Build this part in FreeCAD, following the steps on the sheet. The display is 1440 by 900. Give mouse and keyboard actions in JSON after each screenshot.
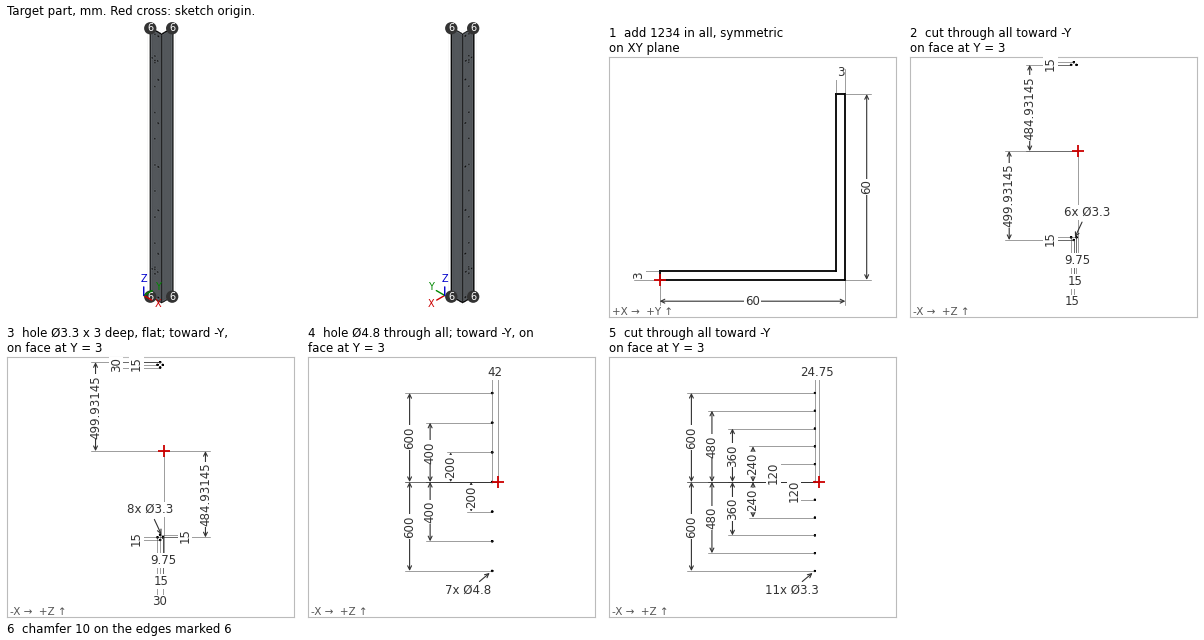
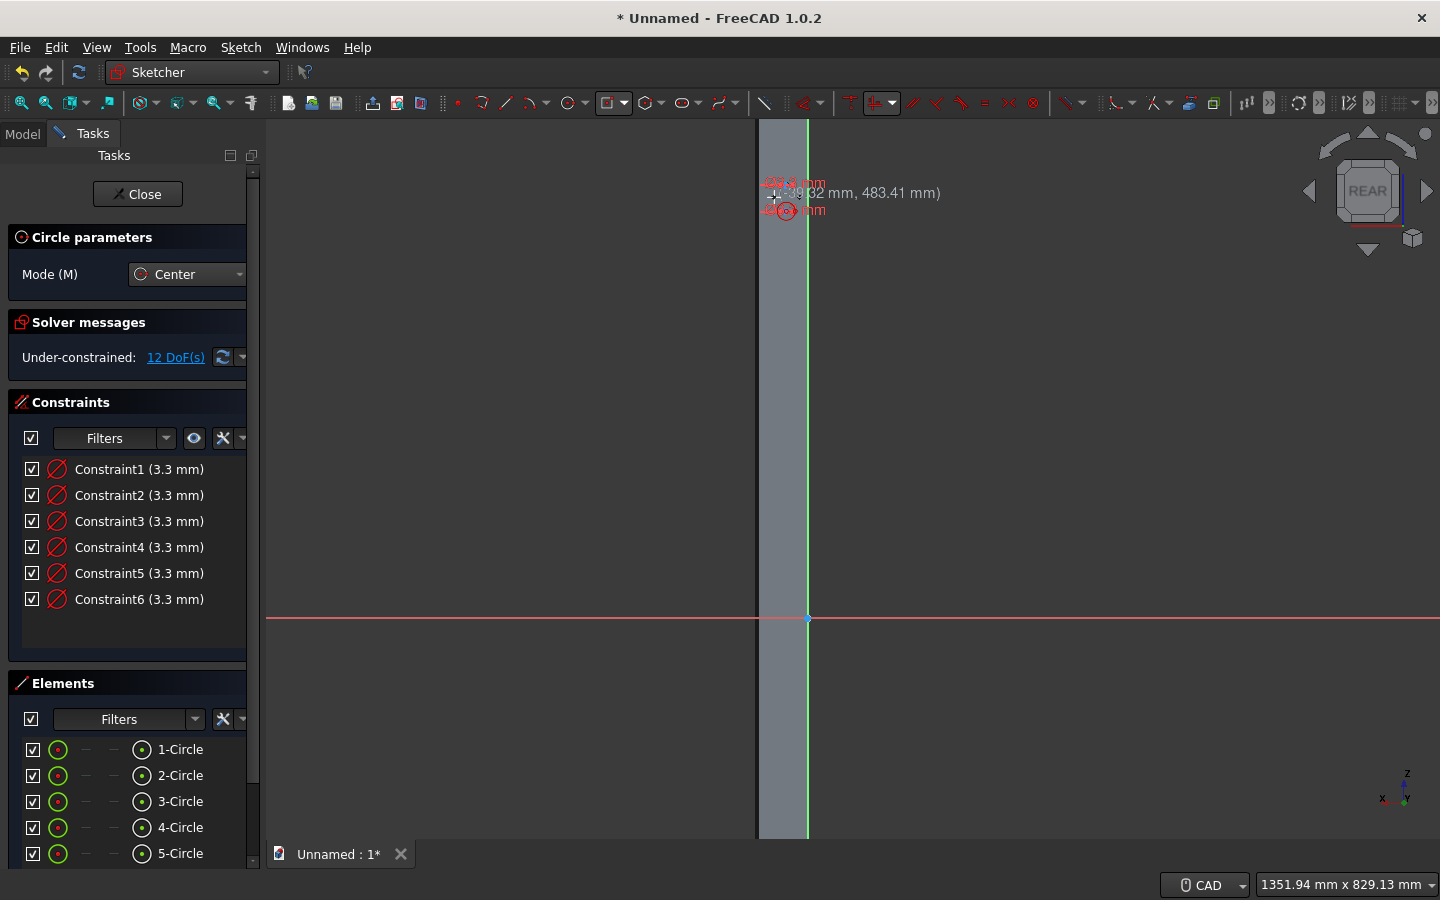
{"action": "left_click", "coordinate": [773, 197]}
{"action": "mouse_move", "coordinate": [774, 196]}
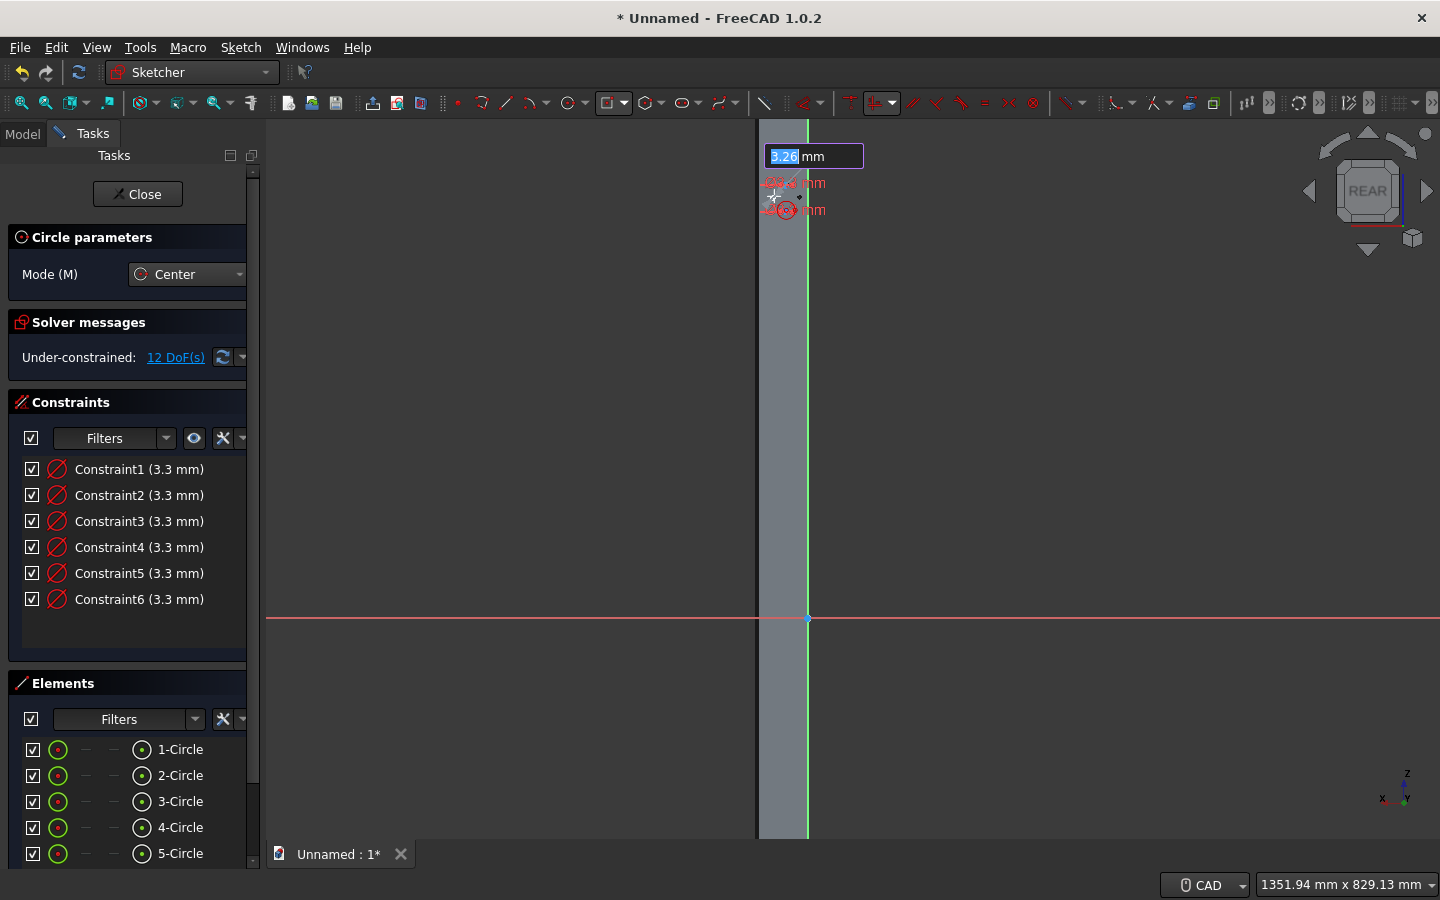
{"action": "type", "text": "3.3"}
{"action": "key", "text": "Return"}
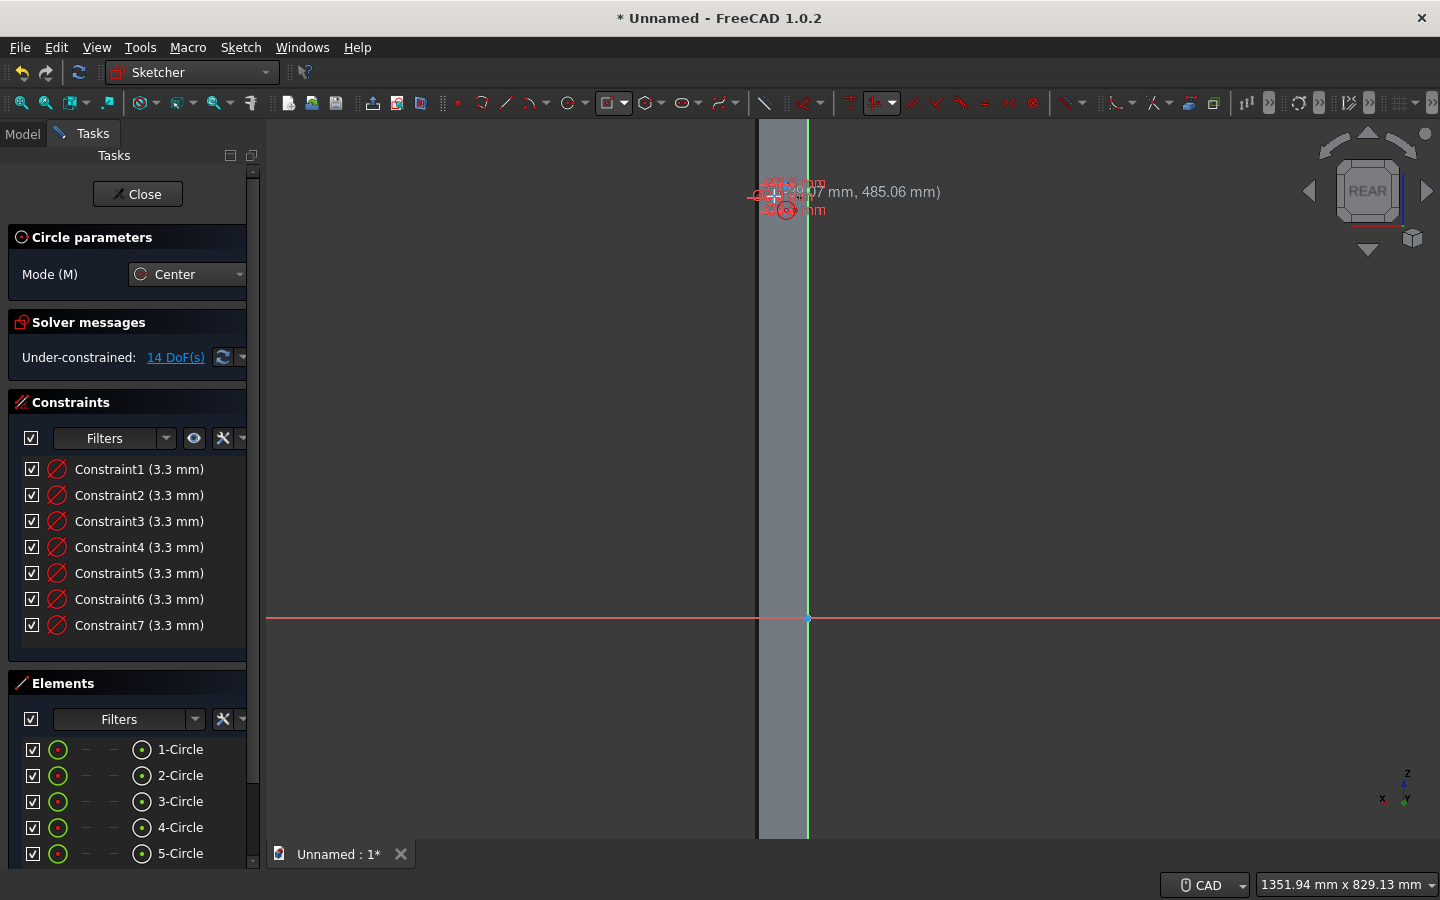
{"action": "scroll", "coordinate": [799, 197], "scroll_direction": "up", "scroll_amount": 14}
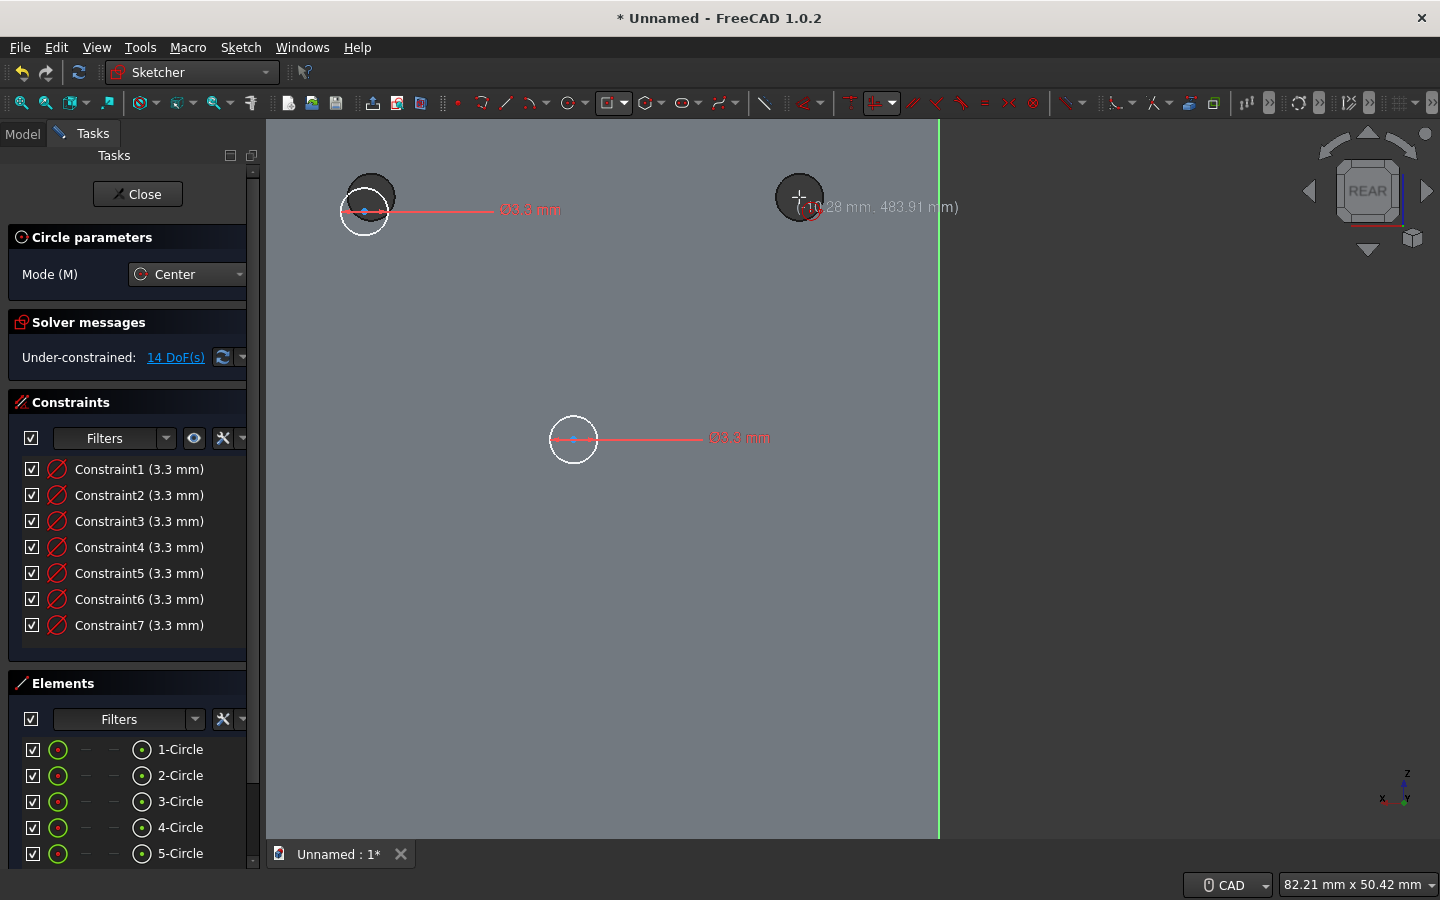
{"action": "scroll", "coordinate": [791, 197], "scroll_direction": "down", "scroll_amount": 16}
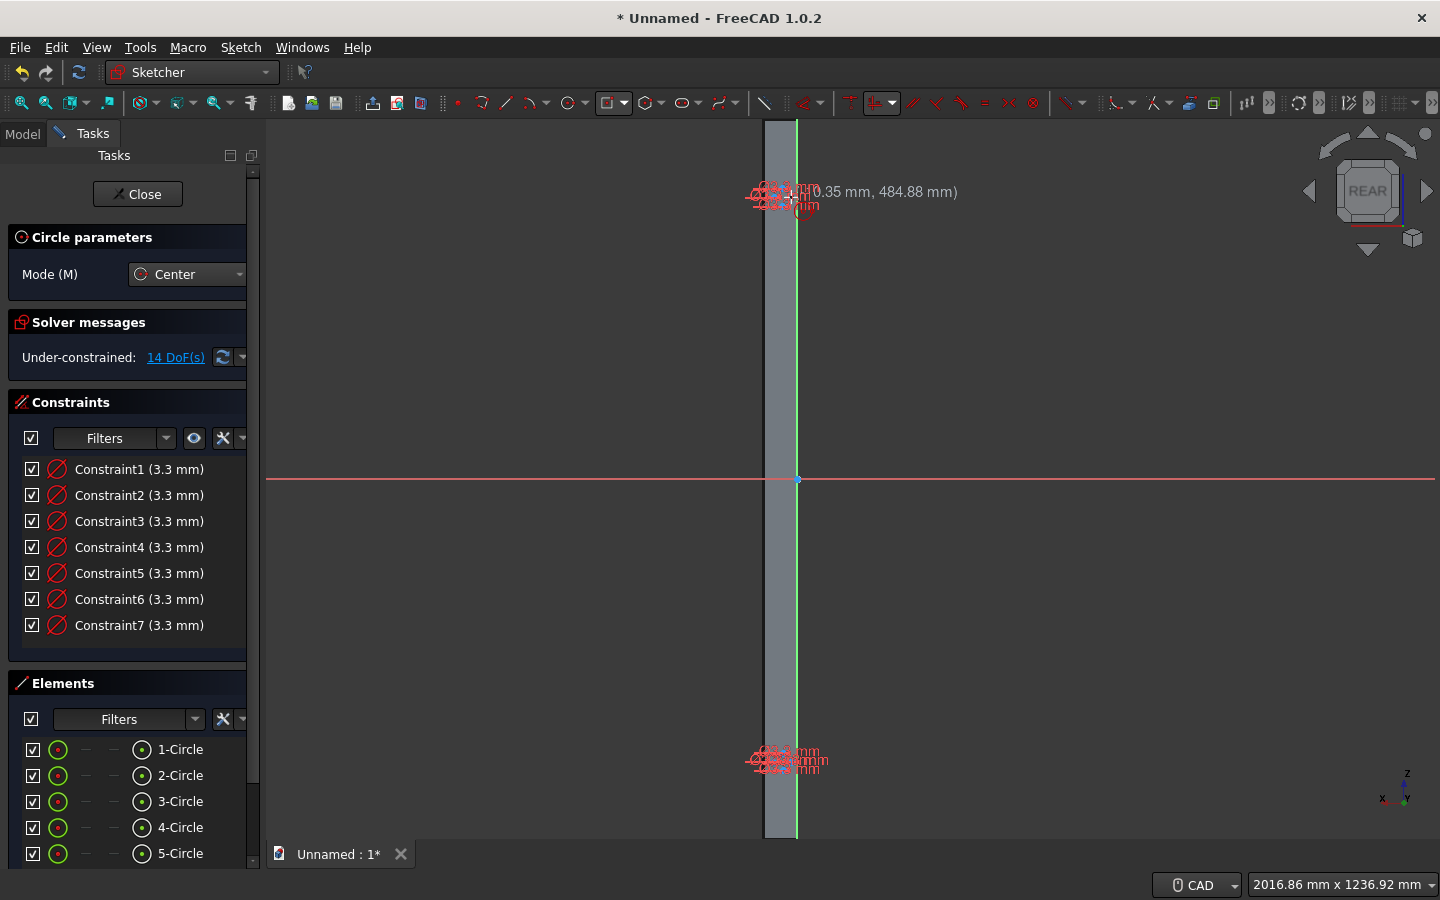
{"action": "scroll", "coordinate": [792, 197], "scroll_direction": "up", "scroll_amount": 6}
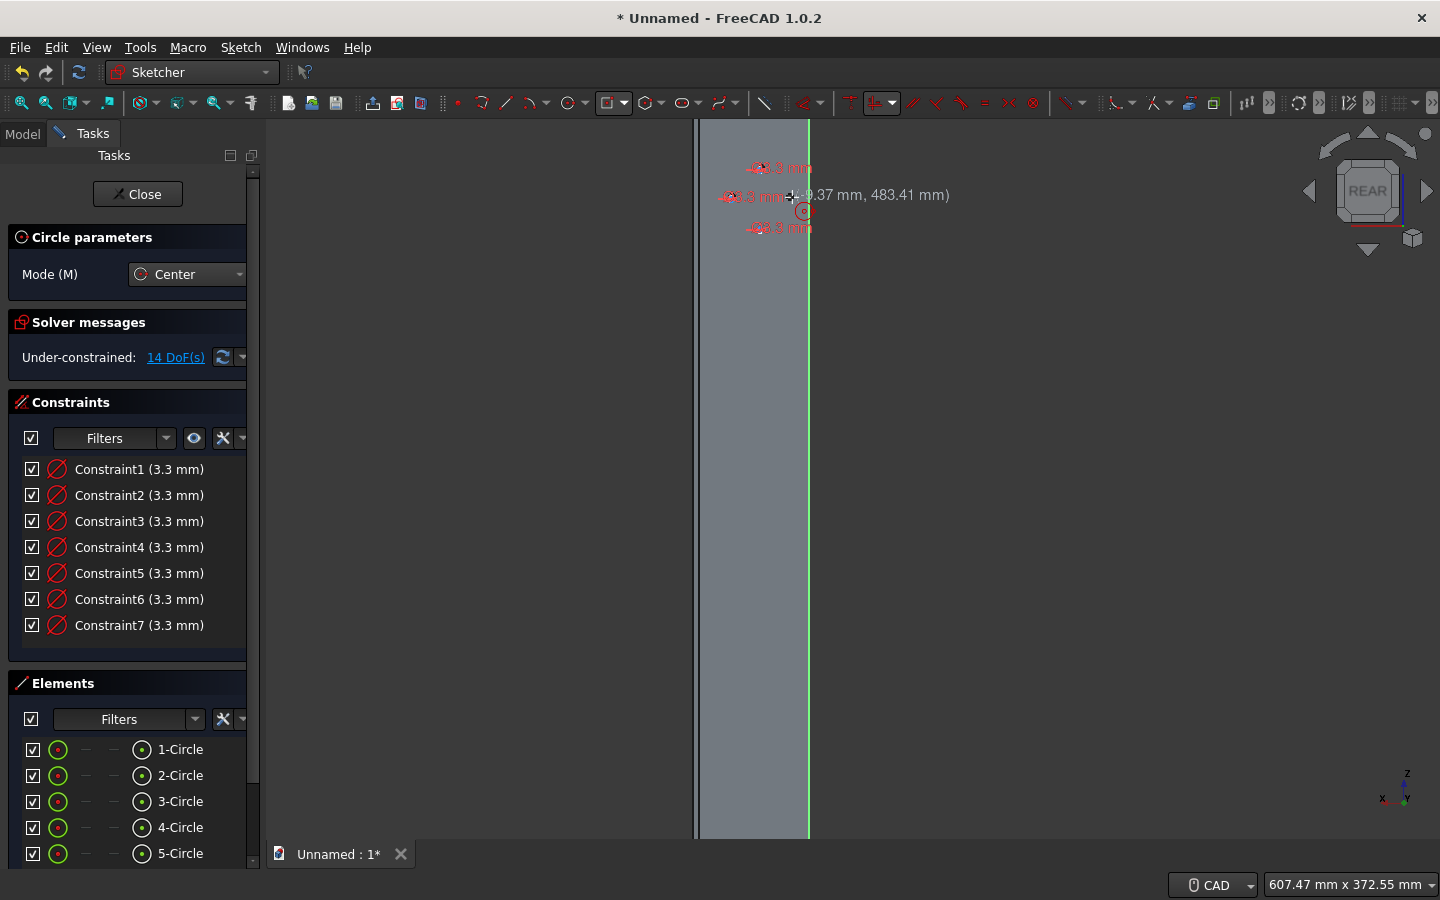
{"action": "left_click", "coordinate": [790, 197]}
{"action": "mouse_move", "coordinate": [792, 195]}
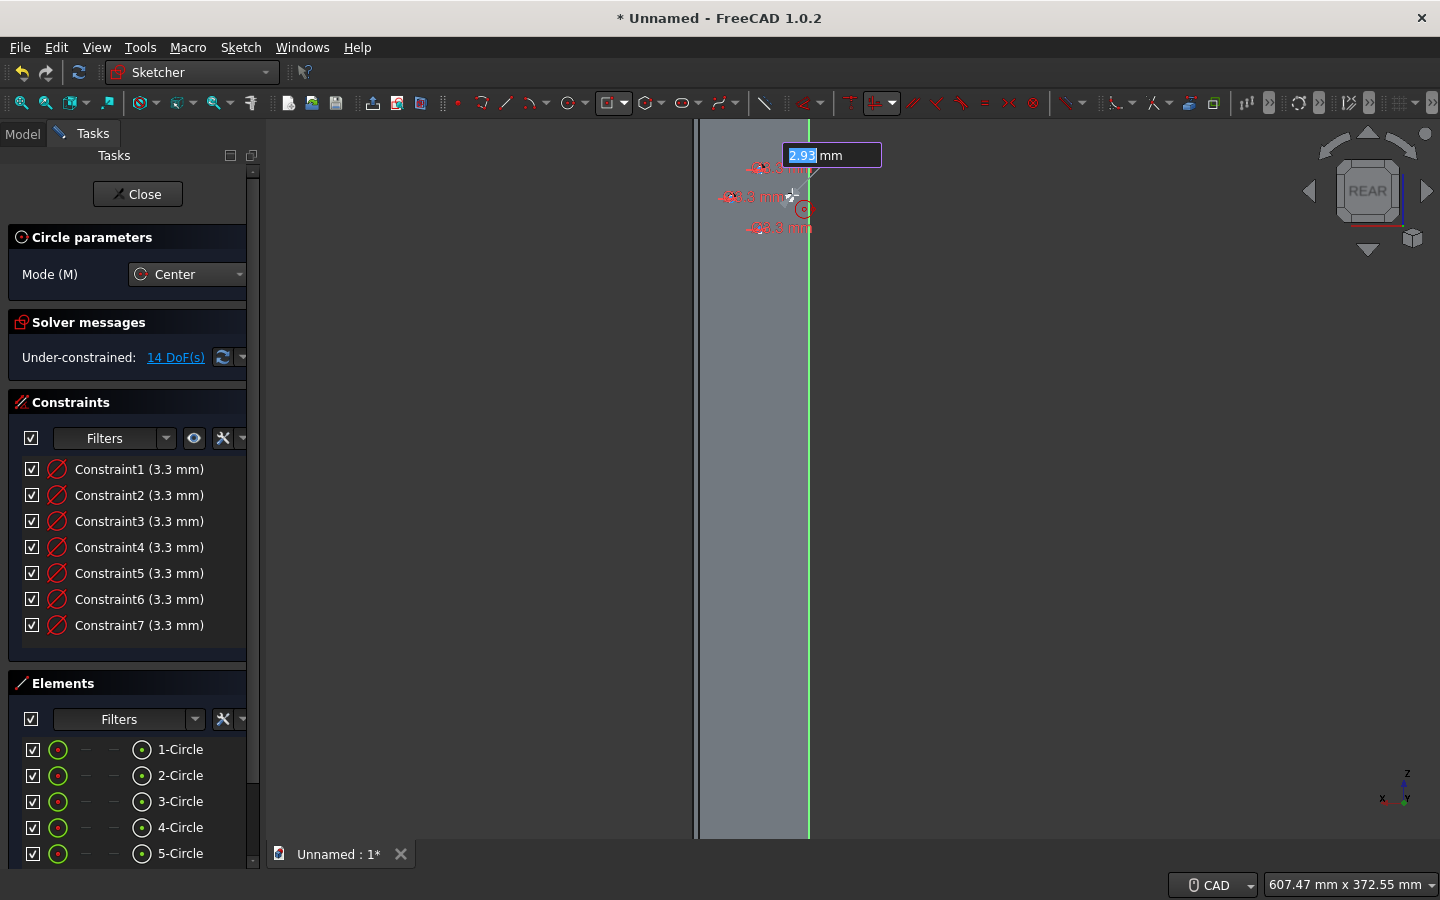
{"action": "type", "text": "3.3"}
{"action": "key", "text": "Return"}
{"action": "key", "text": "Escape"}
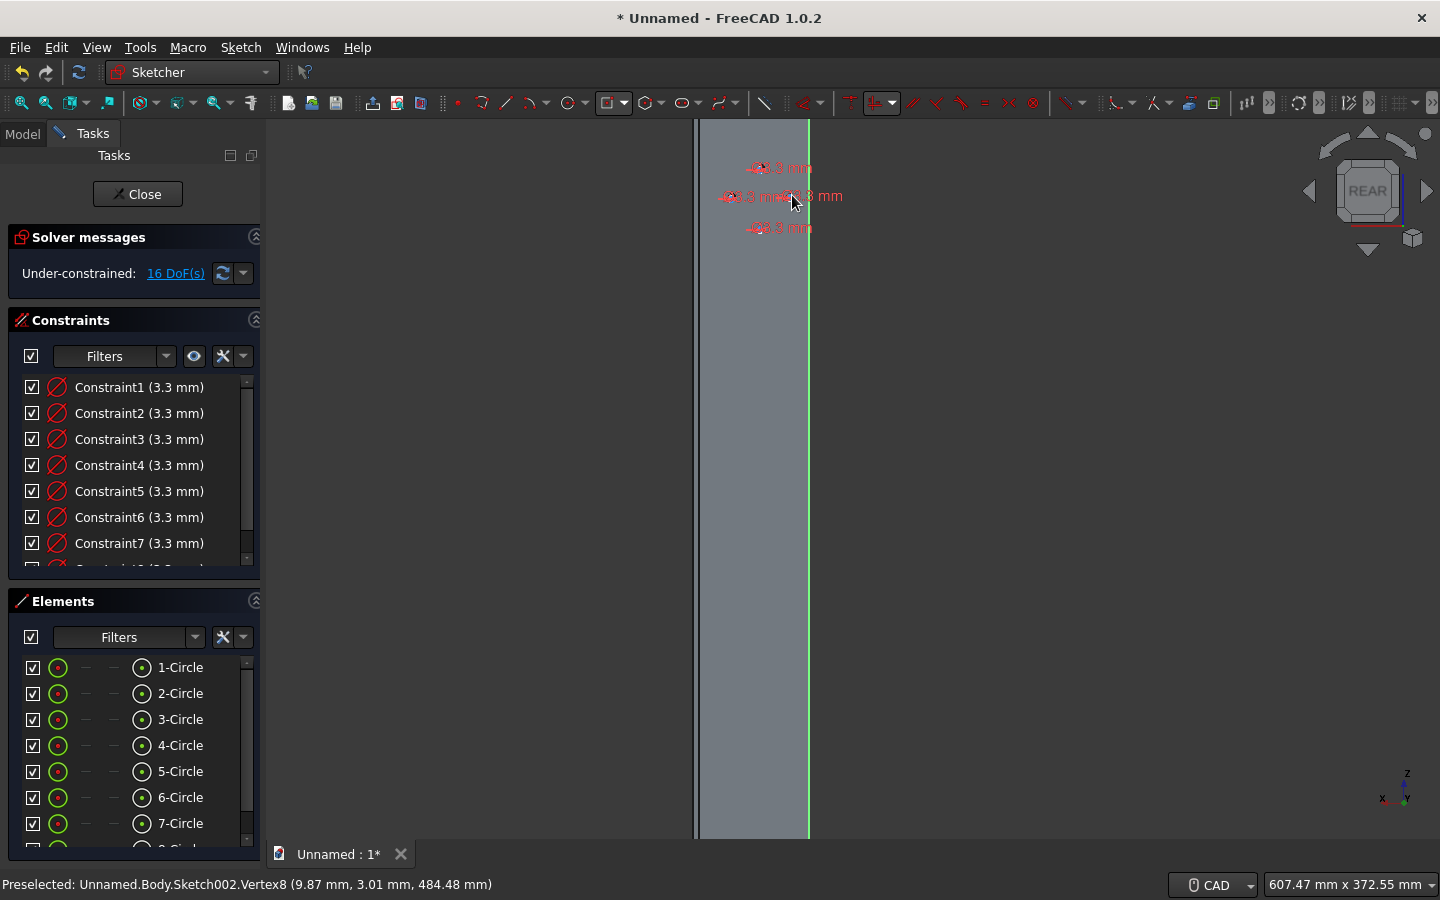
{"action": "scroll", "coordinate": [790, 265], "scroll_direction": "down", "scroll_amount": 7}